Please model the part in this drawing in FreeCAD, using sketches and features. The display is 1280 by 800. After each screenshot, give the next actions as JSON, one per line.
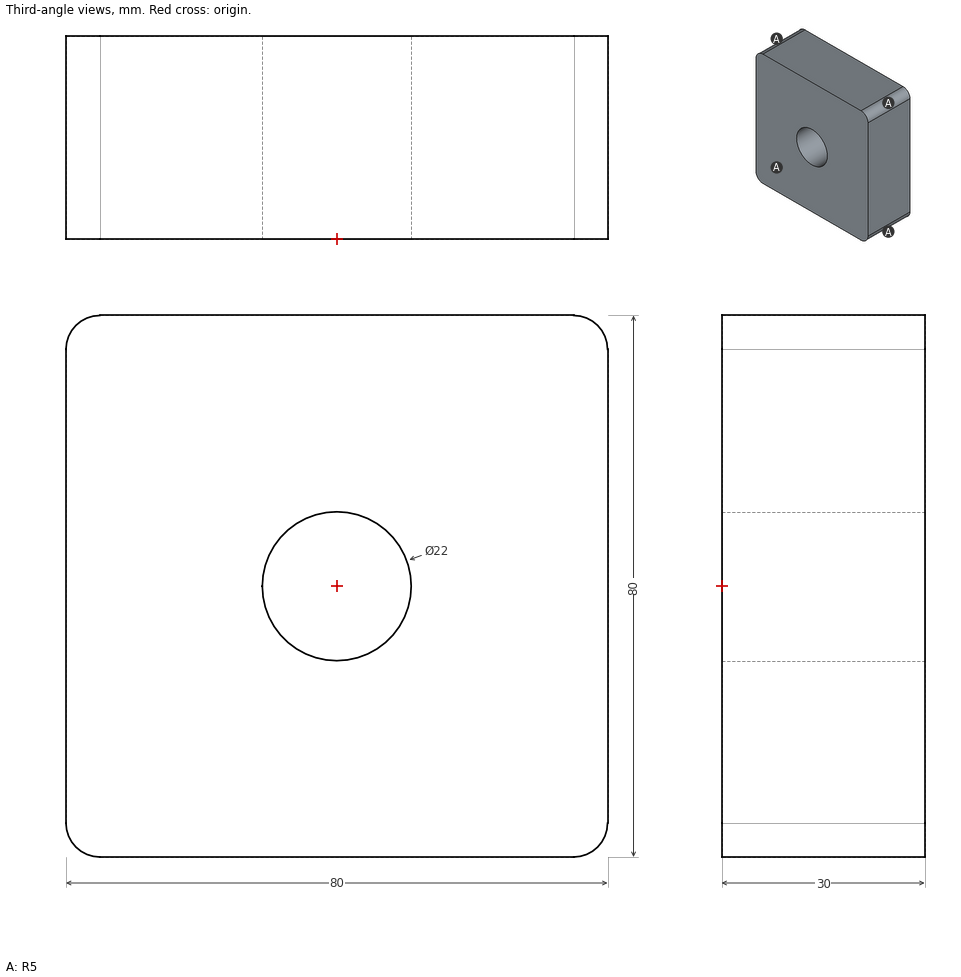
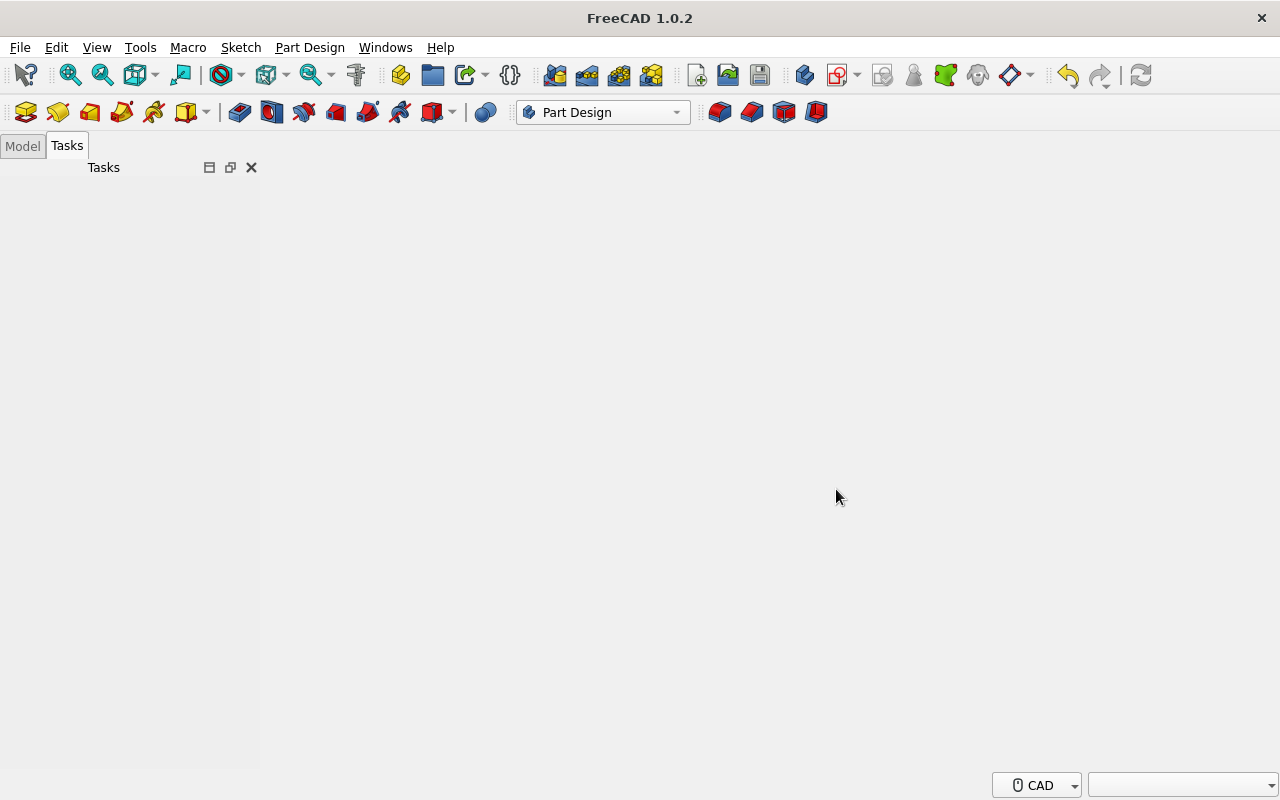
{"action": "left_click", "coordinate": [696, 76]}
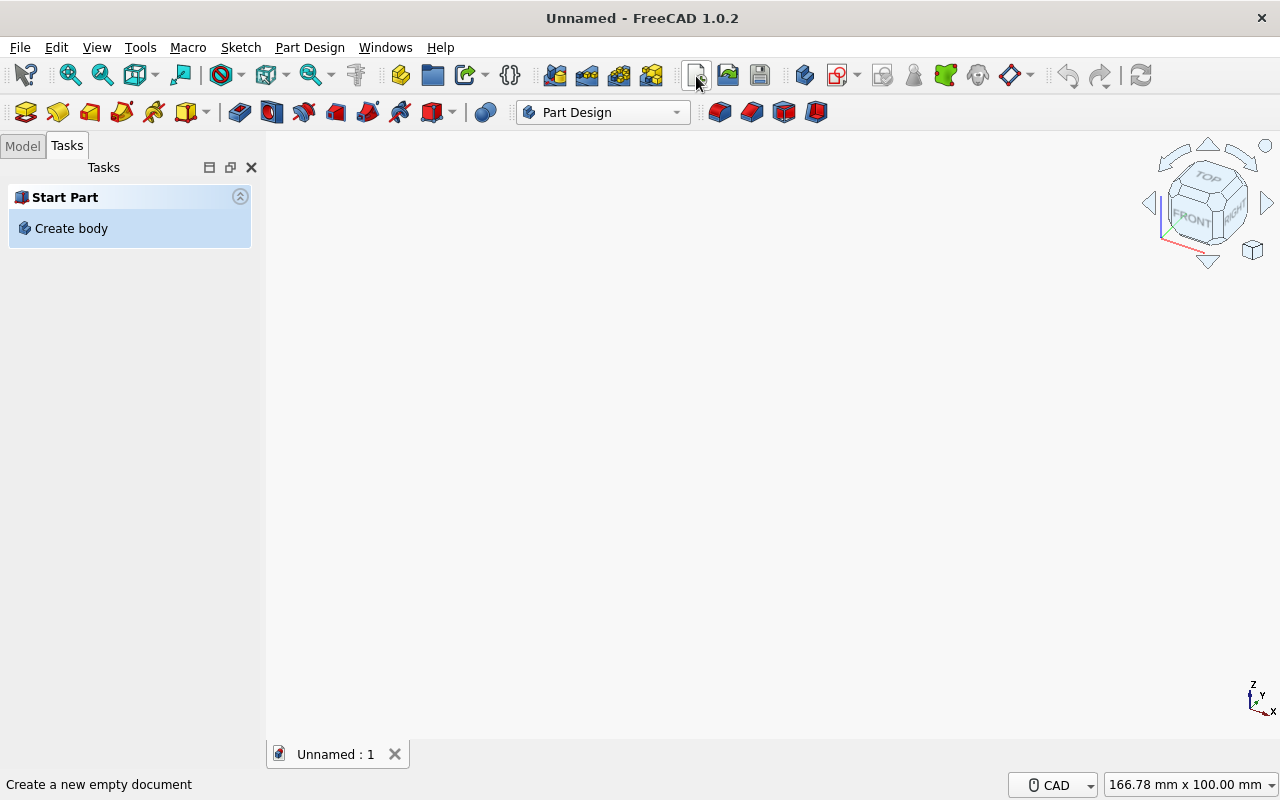
{"action": "left_click", "coordinate": [838, 76]}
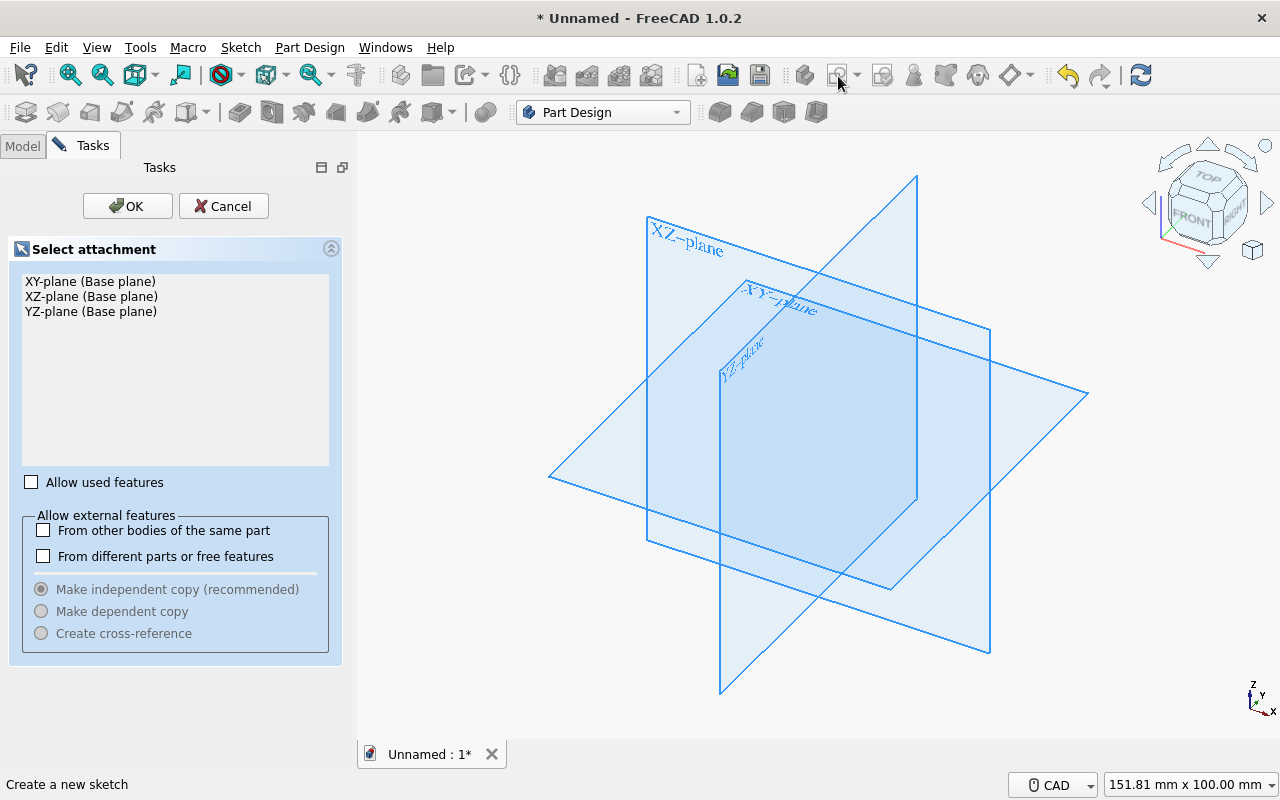
{"action": "left_click", "coordinate": [82, 296]}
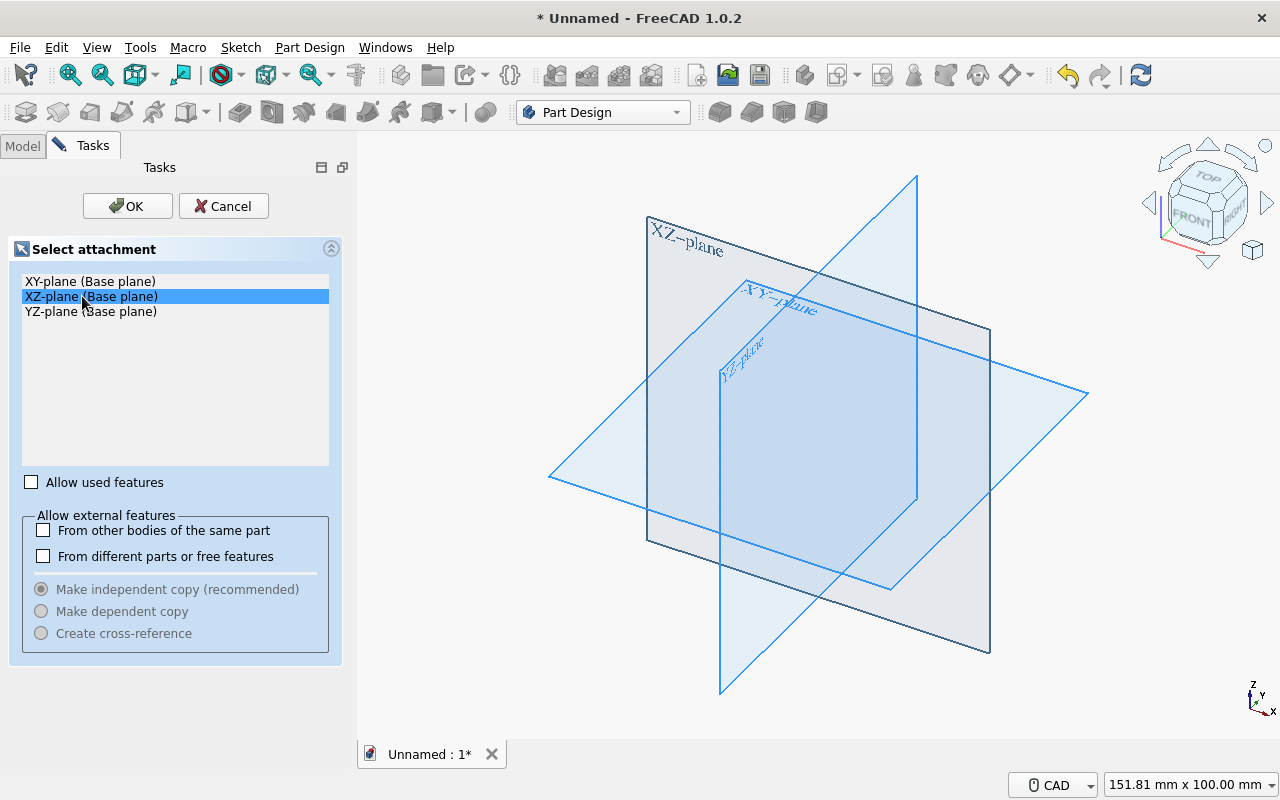
{"action": "left_click", "coordinate": [128, 206]}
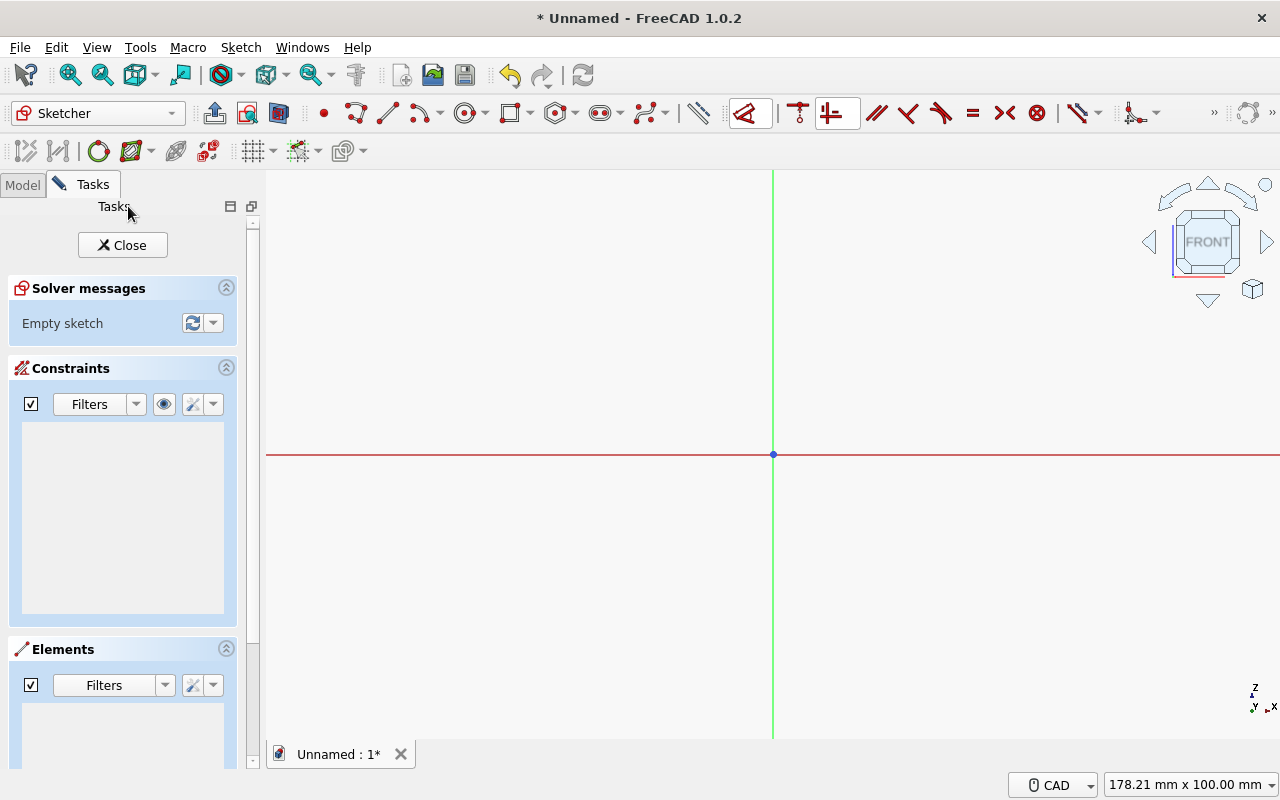
{"action": "left_click", "coordinate": [532, 114]}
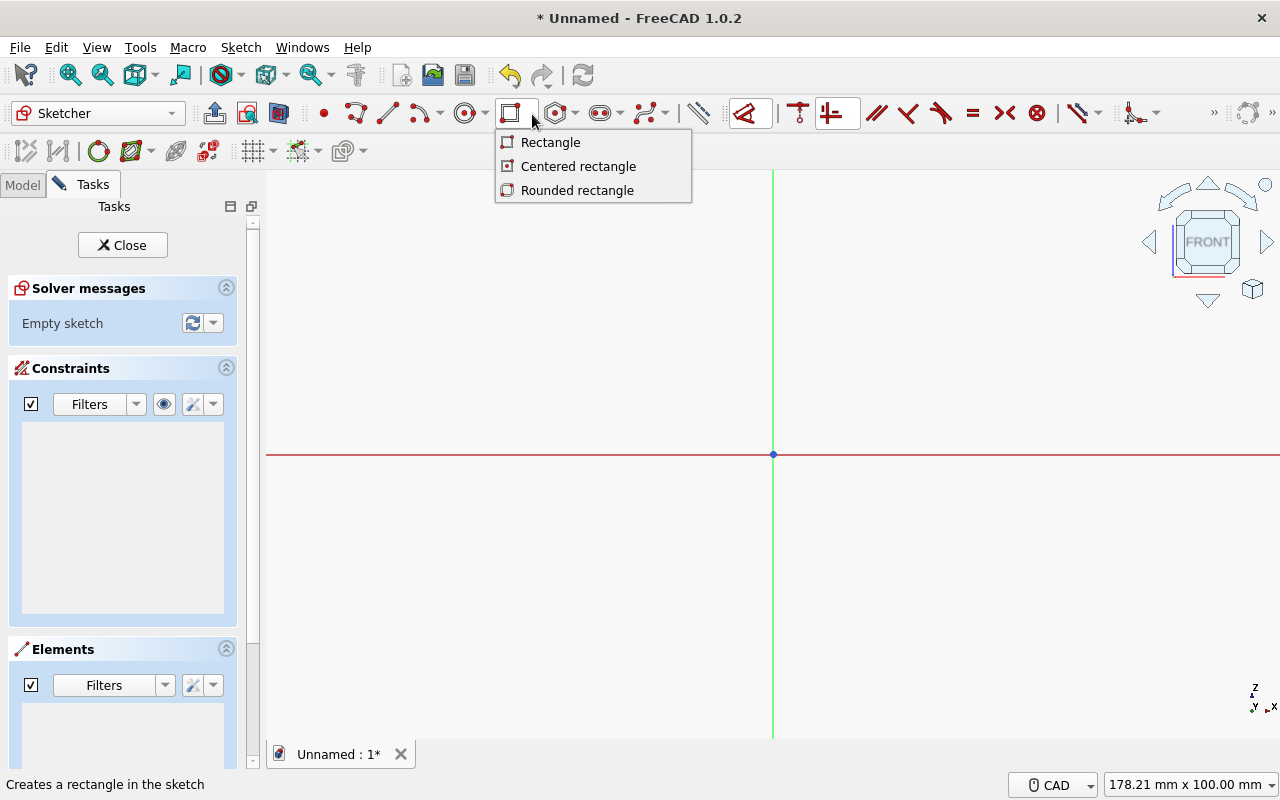
{"action": "left_click", "coordinate": [594, 166]}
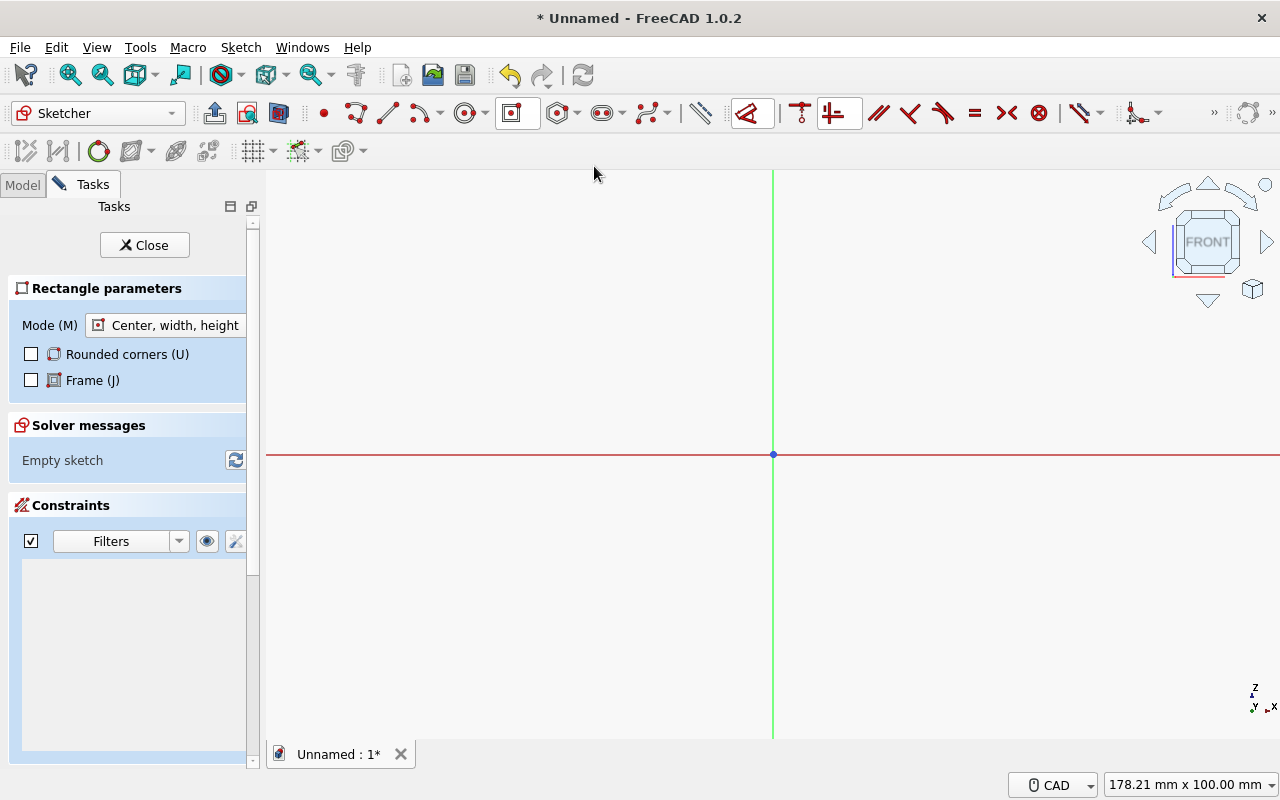
{"action": "left_click", "coordinate": [773, 454]}
{"action": "left_click", "coordinate": [1001, 227]}
{"action": "key", "text": "Escape"}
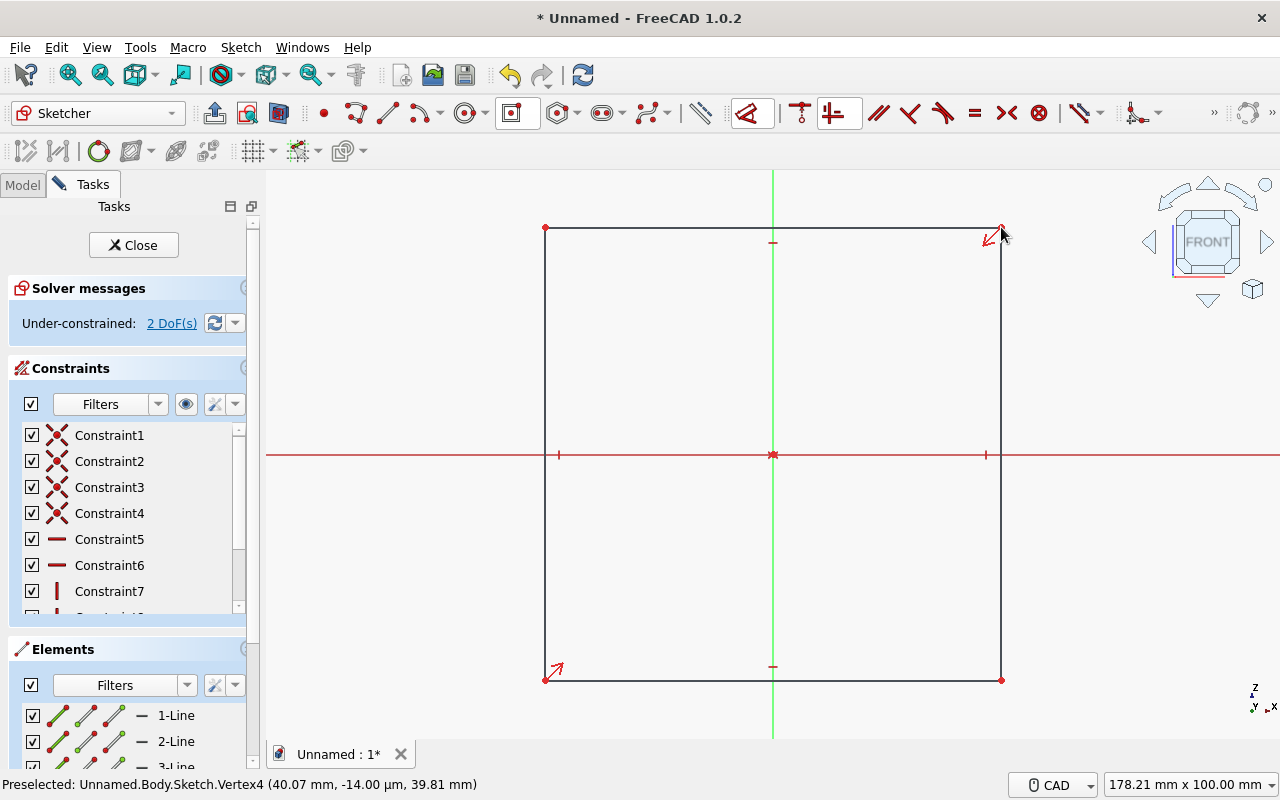
{"action": "left_click", "coordinate": [746, 114]}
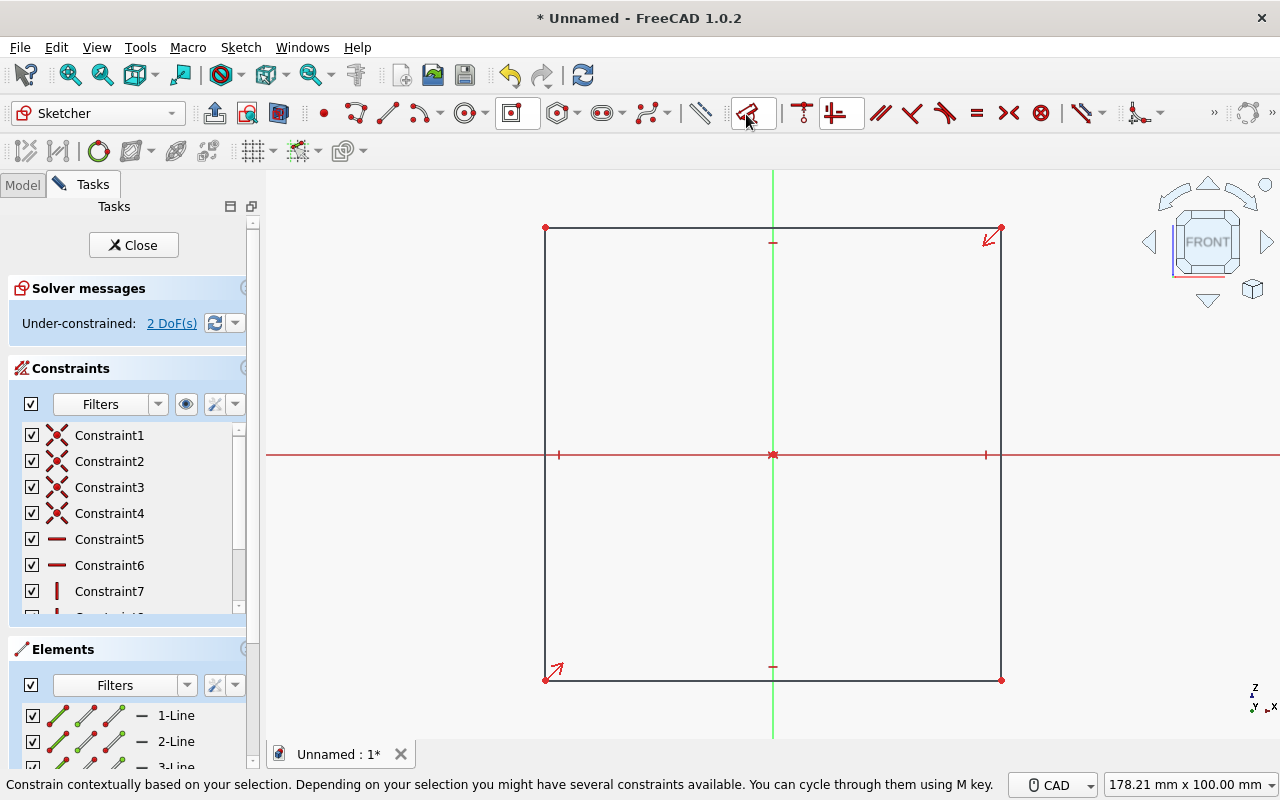
{"action": "left_click", "coordinate": [682, 681]}
{"action": "left_click", "coordinate": [668, 647]}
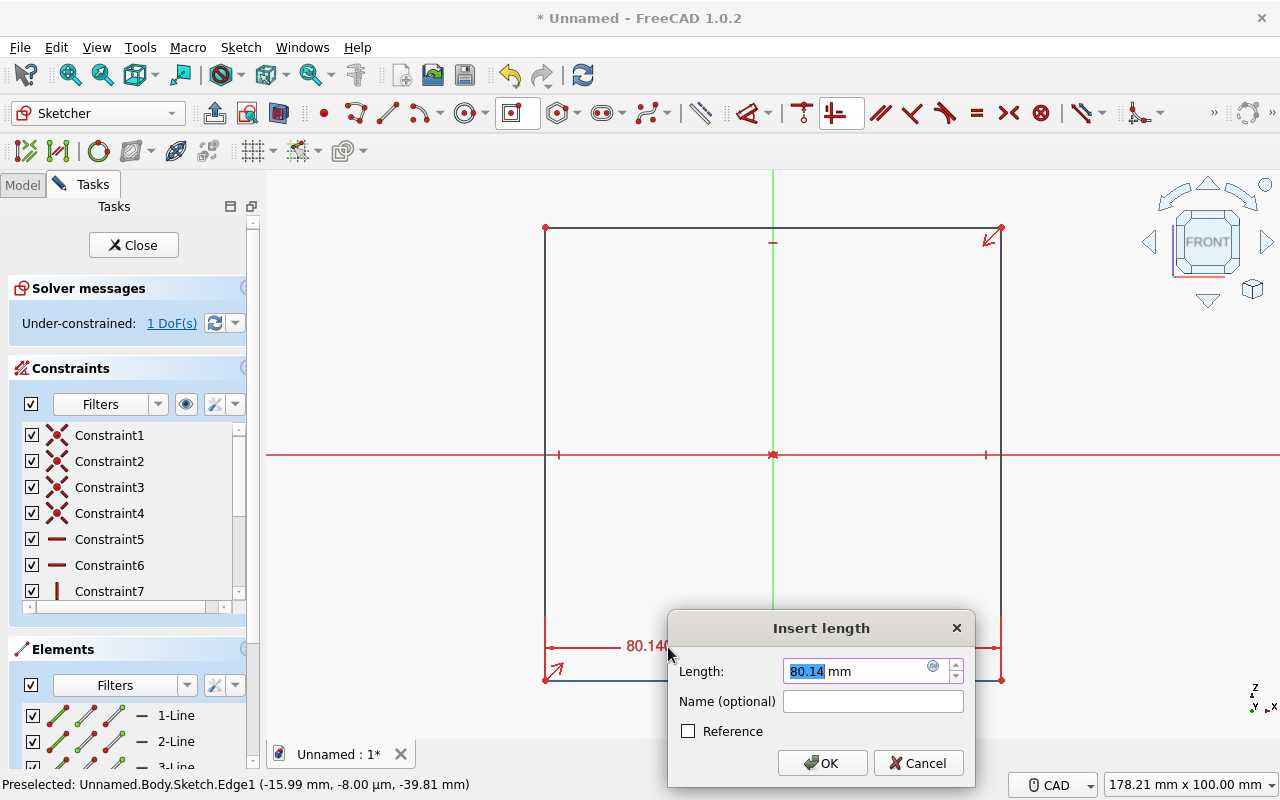
{"action": "type", "text": "80"}
{"action": "key", "text": "Return"}